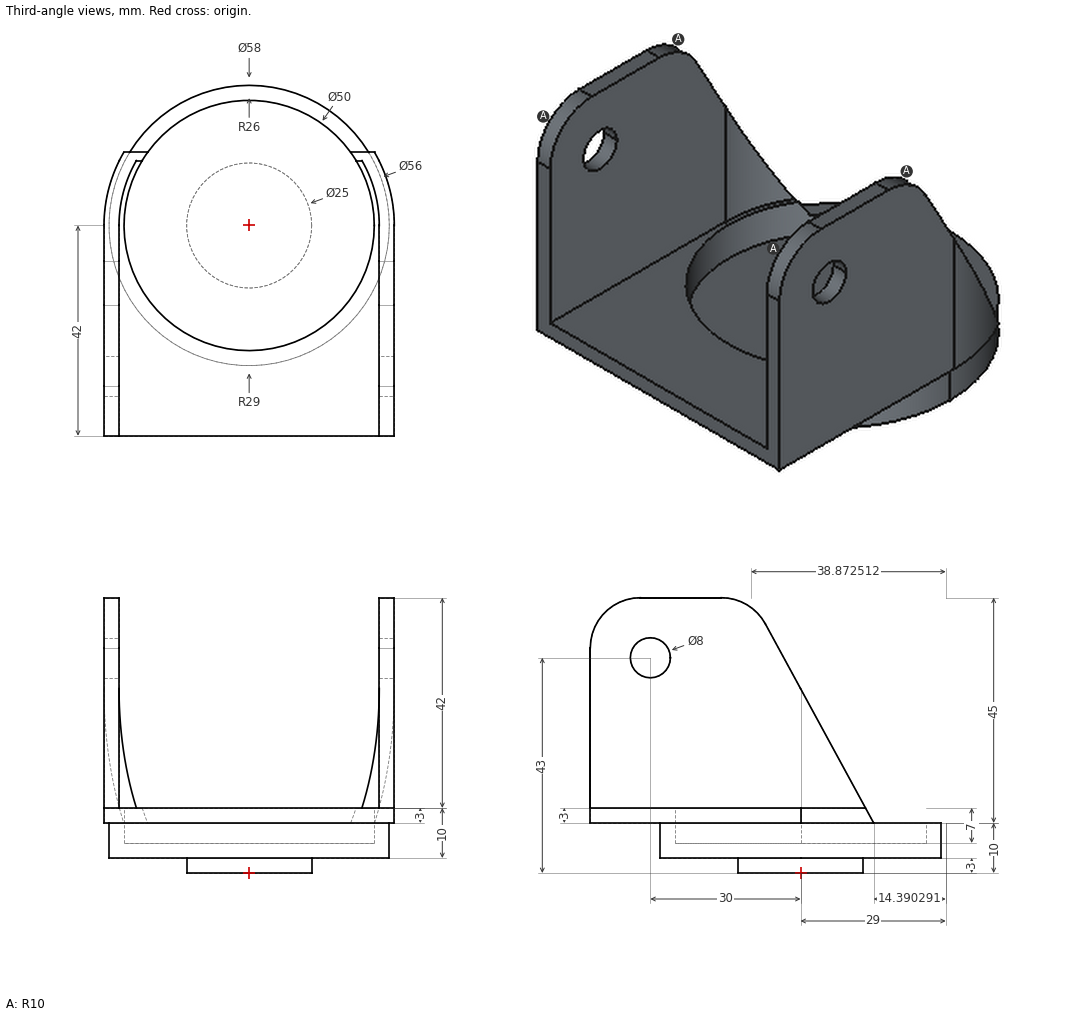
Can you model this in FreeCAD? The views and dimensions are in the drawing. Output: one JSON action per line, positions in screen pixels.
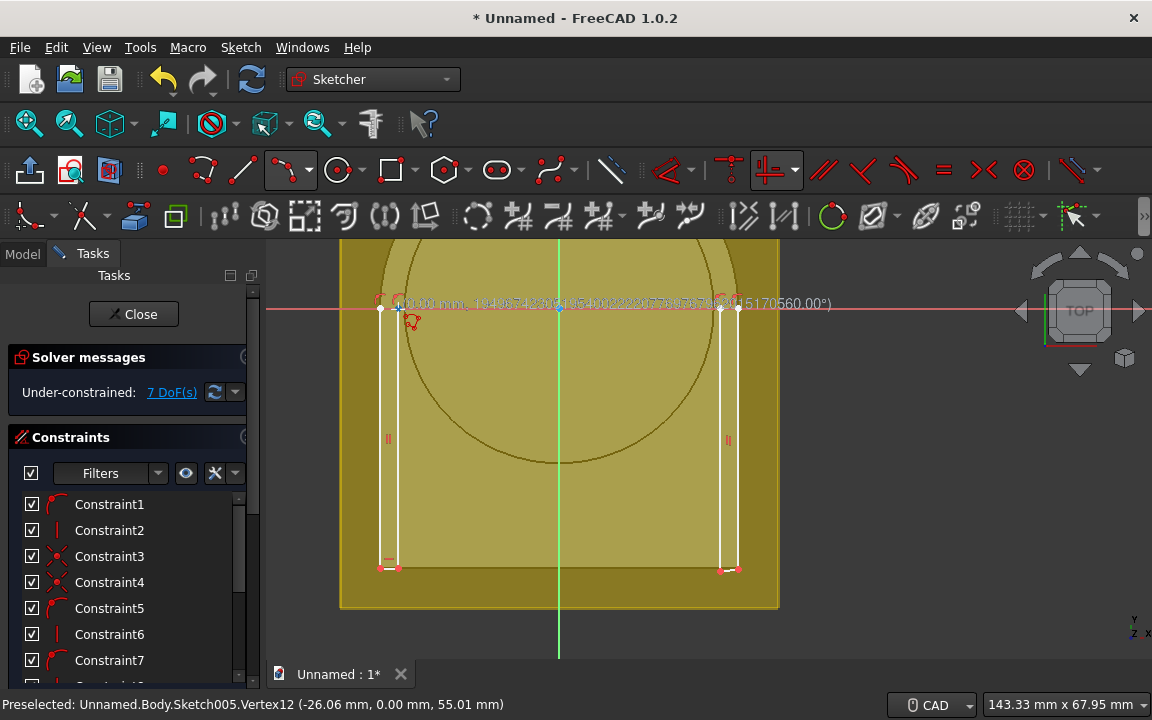
{"action": "left_click", "coordinate": [284, 170]}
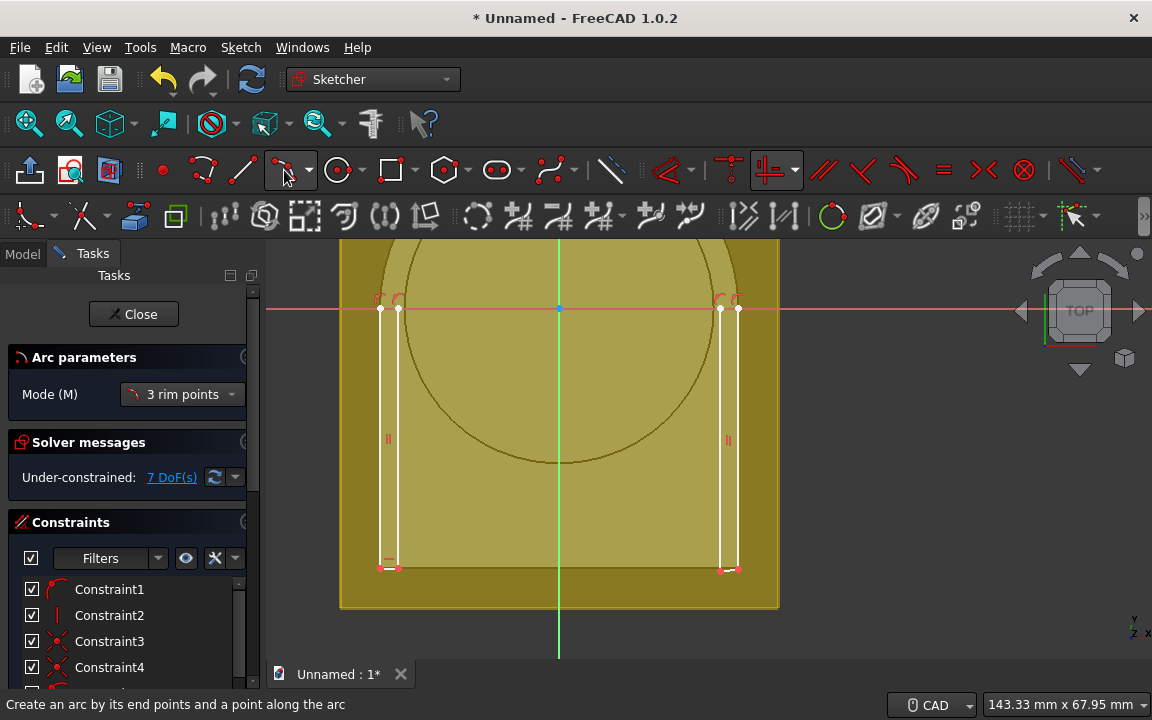
{"action": "left_click", "coordinate": [738, 309]}
{"action": "left_click", "coordinate": [380, 309]}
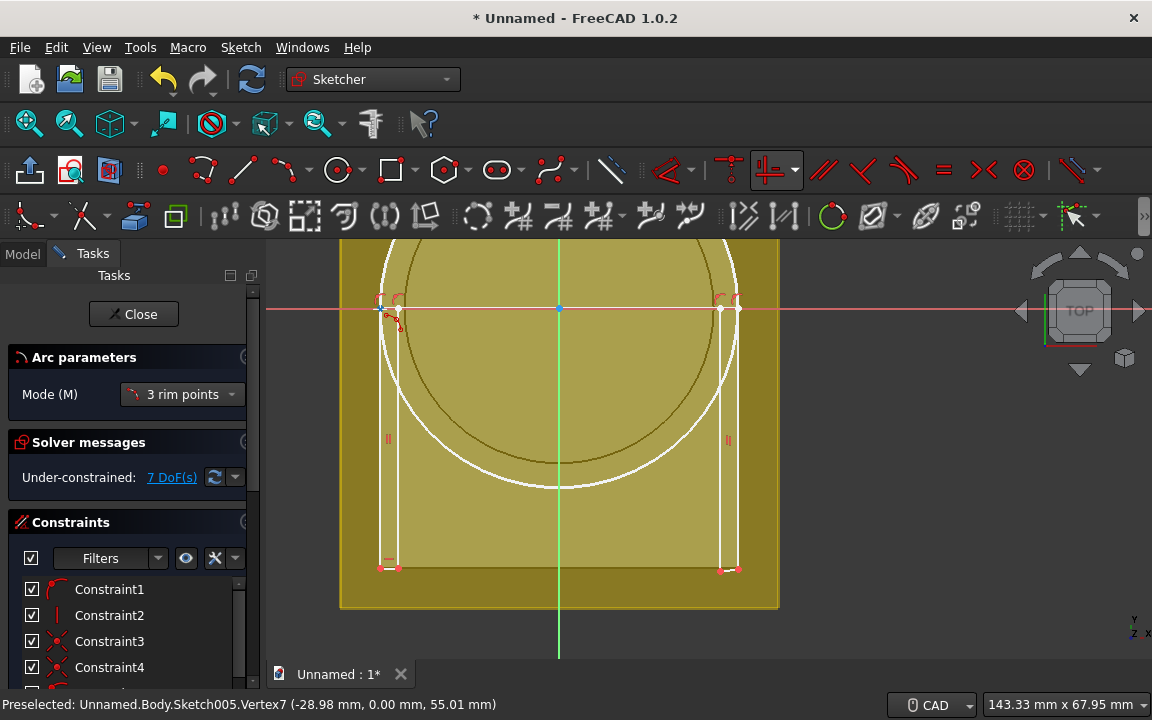
{"action": "scroll", "coordinate": [740, 571], "scroll_direction": "down", "scroll_amount": 3}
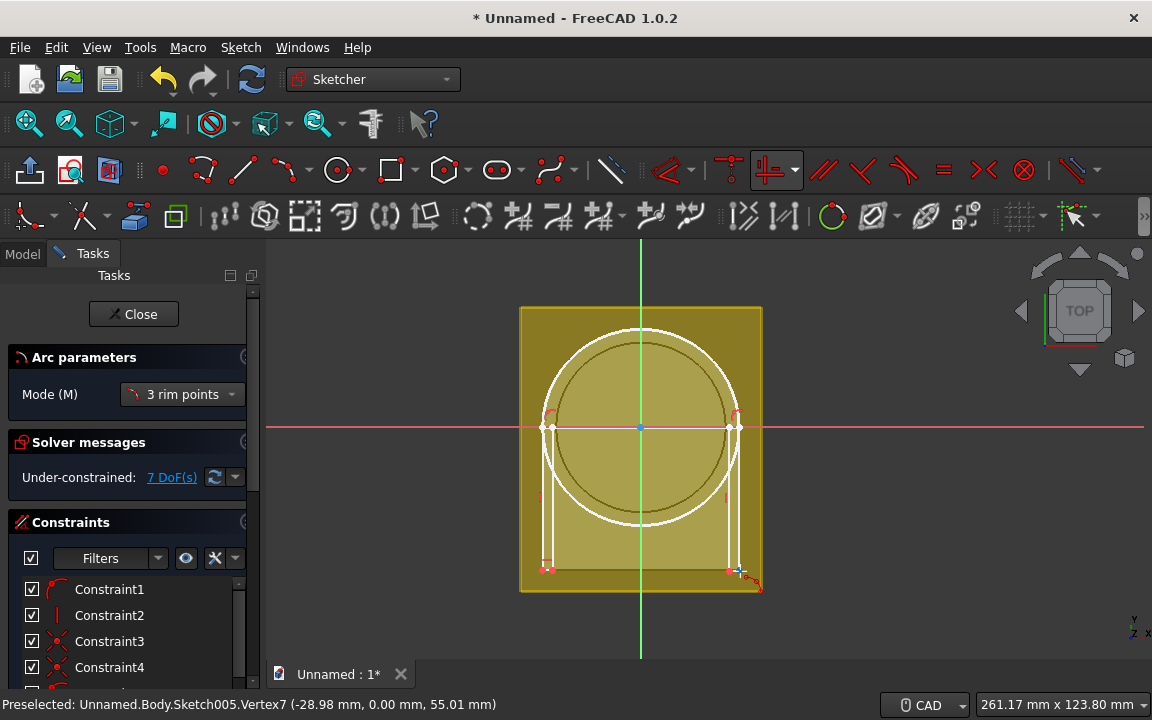
{"action": "left_click", "coordinate": [671, 334]}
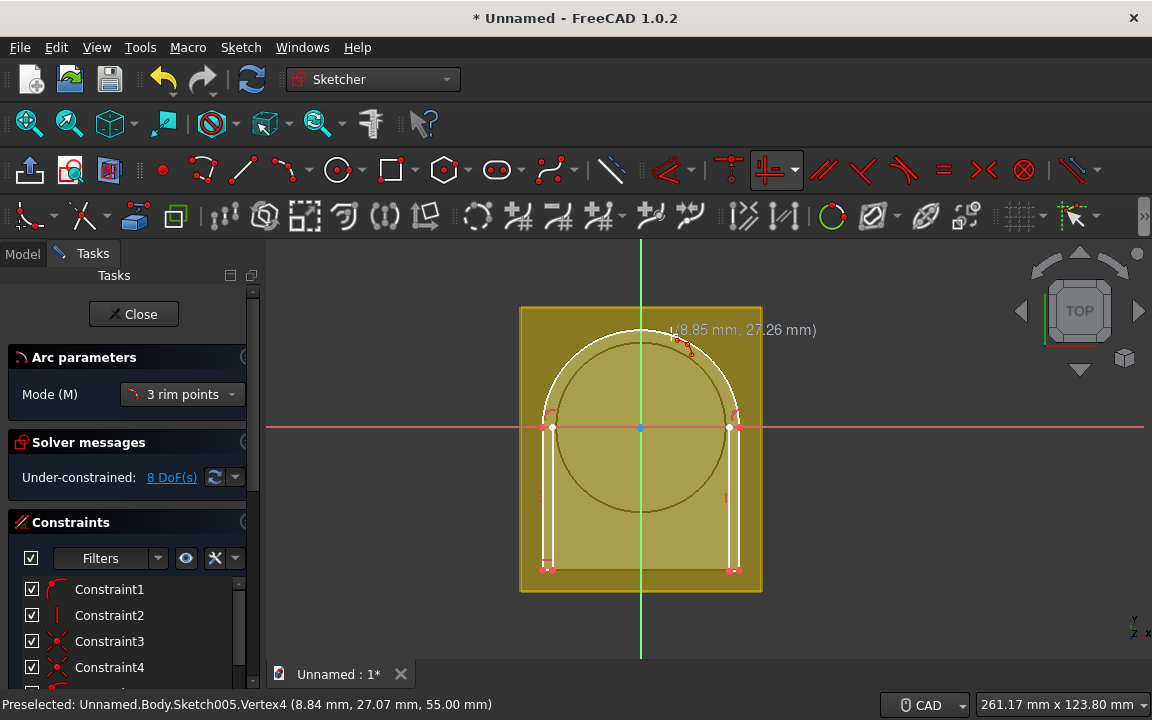
{"action": "scroll", "coordinate": [553, 427], "scroll_direction": "up", "scroll_amount": 3}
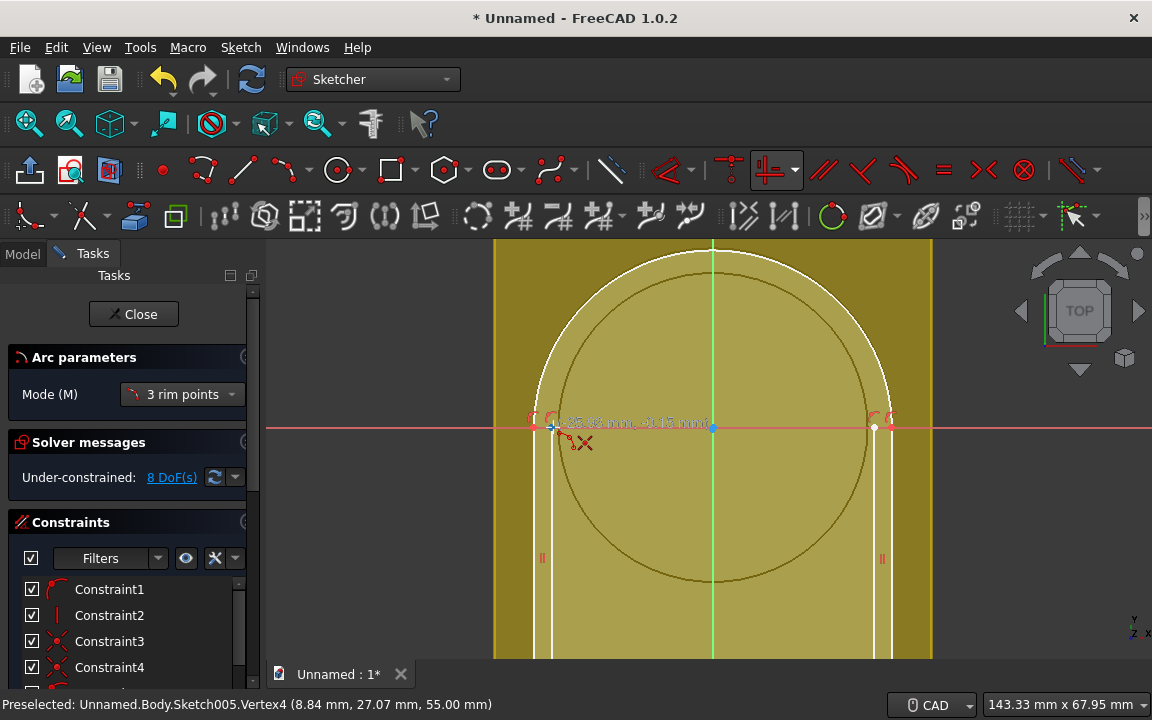
{"action": "left_click", "coordinate": [552, 427]}
{"action": "left_click", "coordinate": [874, 427]}
{"action": "left_click", "coordinate": [619, 297]}
{"action": "key", "text": "Escape"}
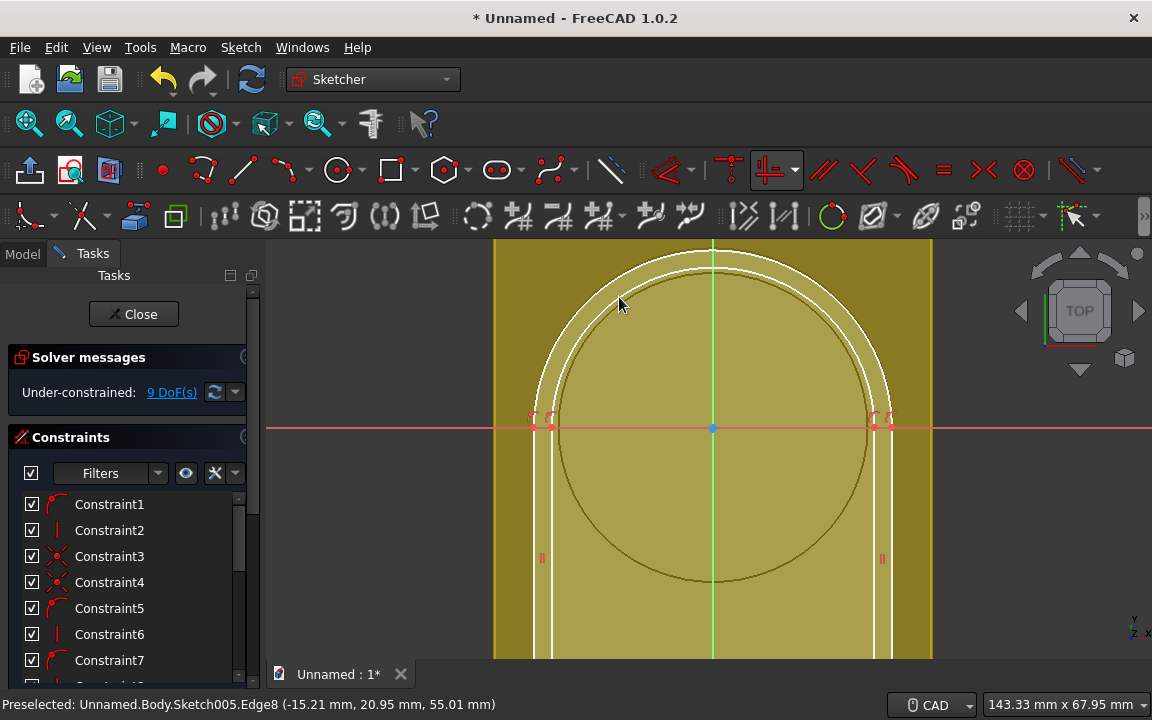
{"action": "left_click", "coordinate": [874, 506]}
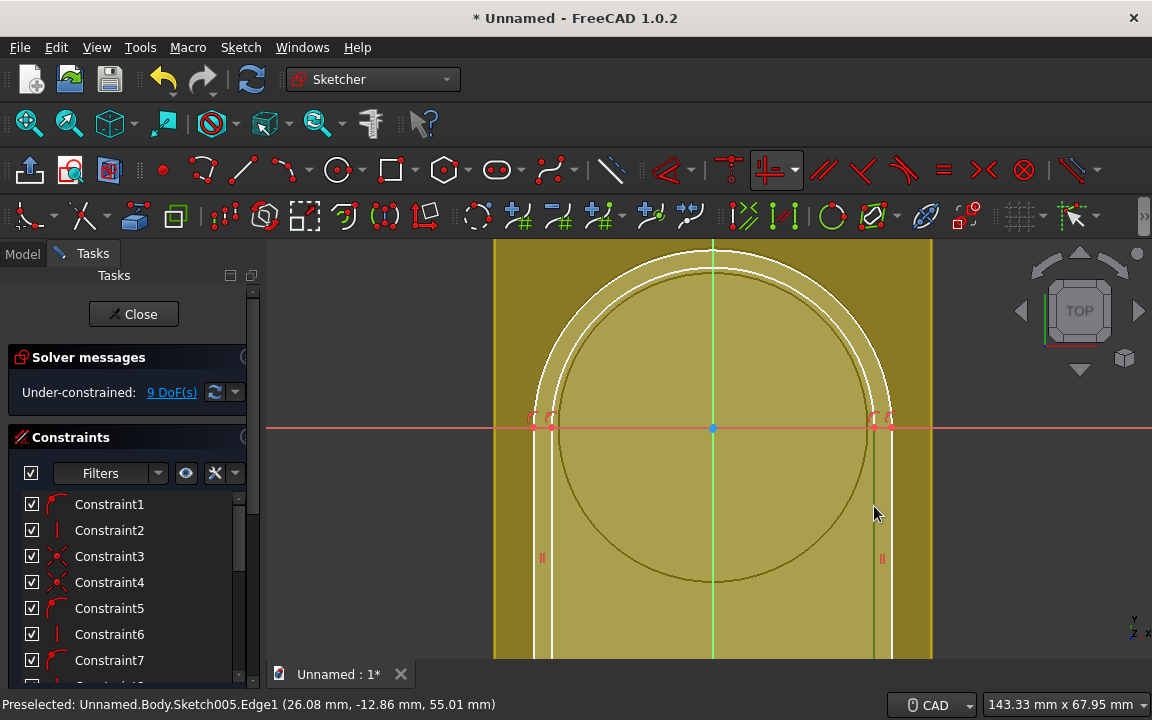
{"action": "left_click", "coordinate": [807, 298]}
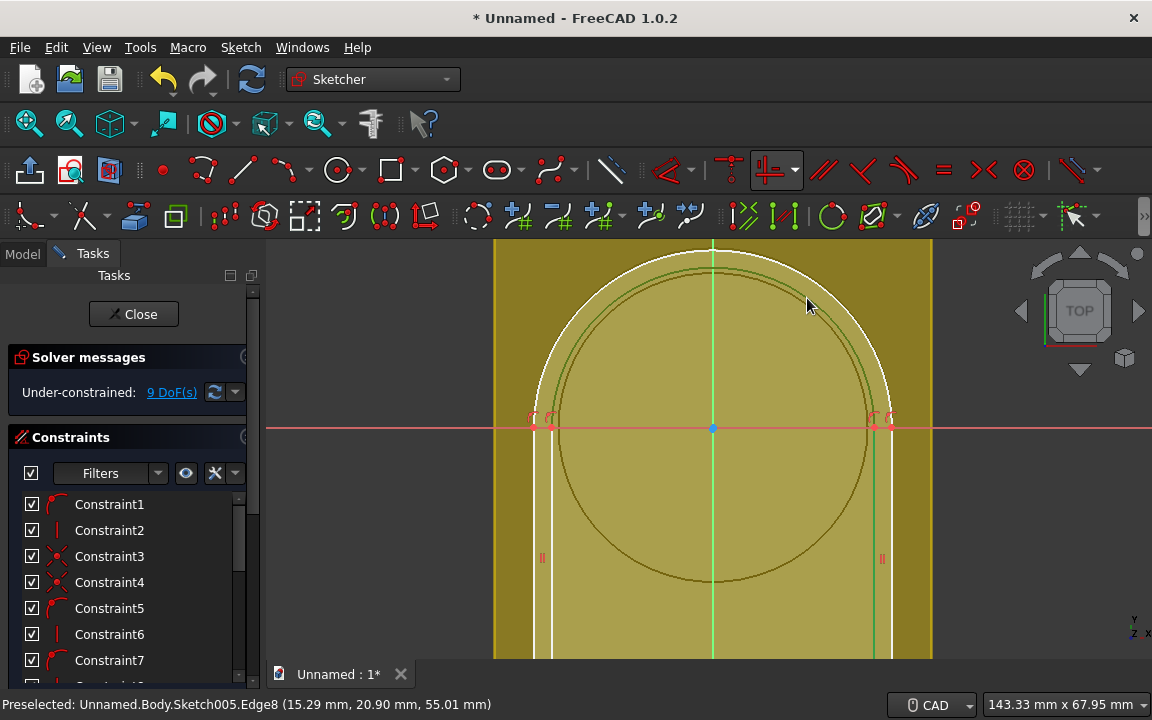
{"action": "left_click", "coordinate": [904, 170]}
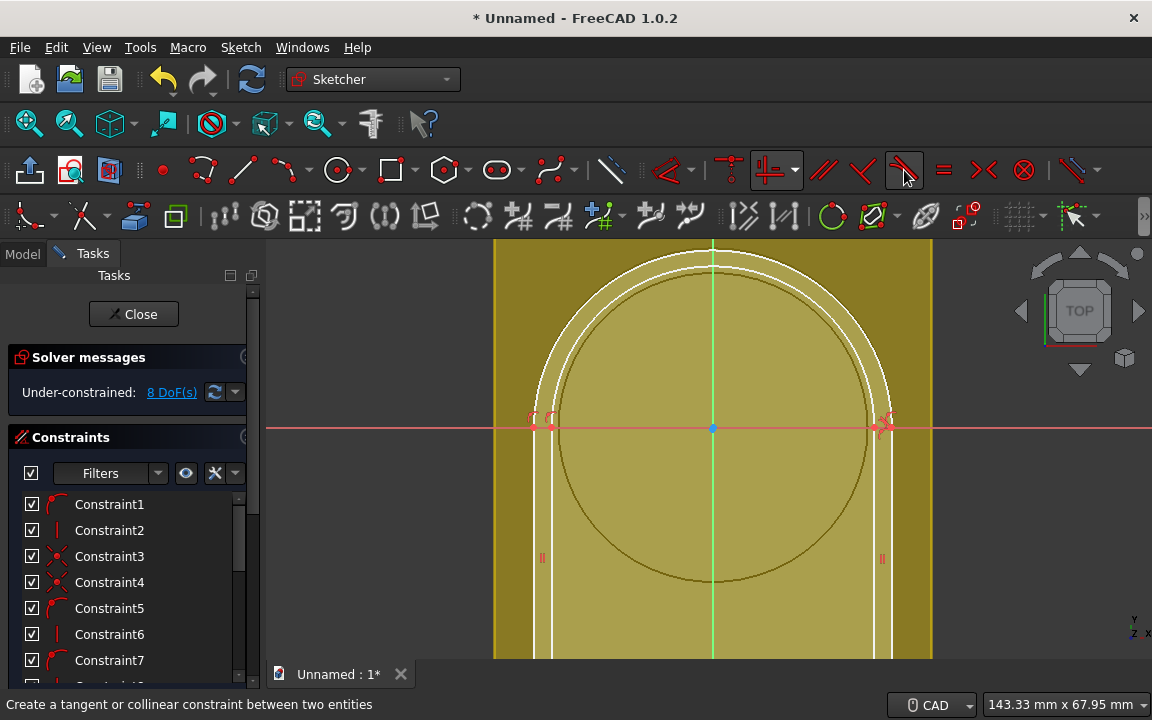
{"action": "scroll", "coordinate": [552, 426], "scroll_direction": "down", "scroll_amount": 3}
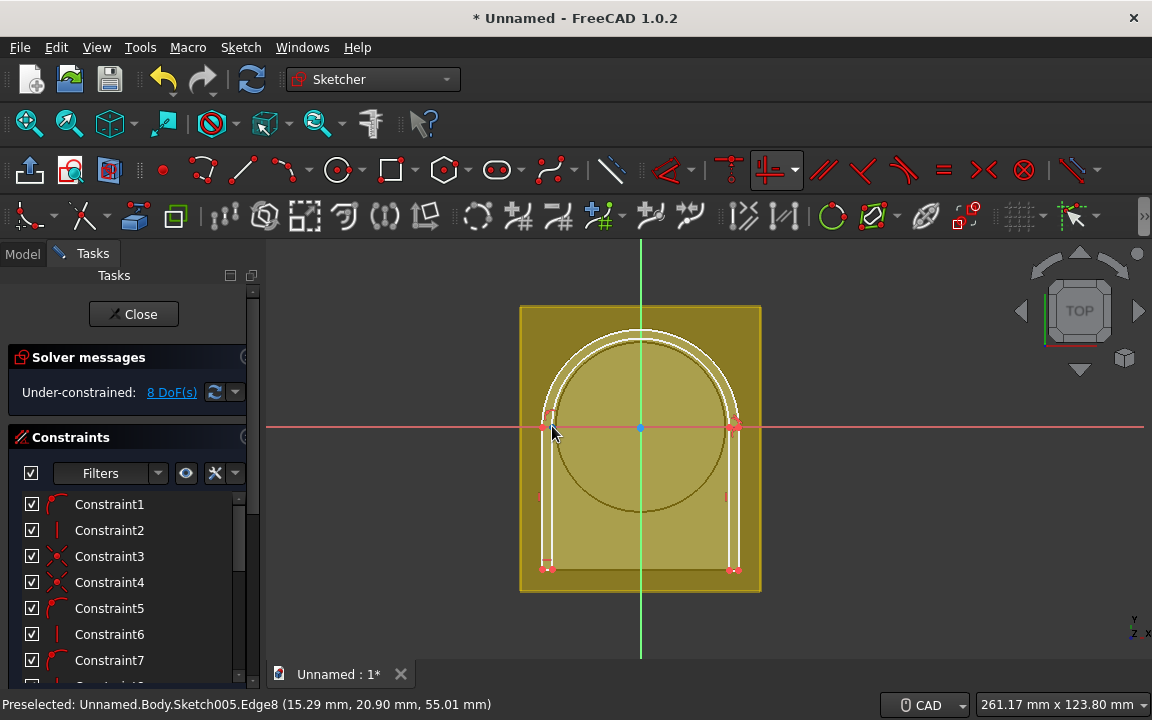
{"action": "scroll", "coordinate": [734, 571], "scroll_direction": "up", "scroll_amount": 6}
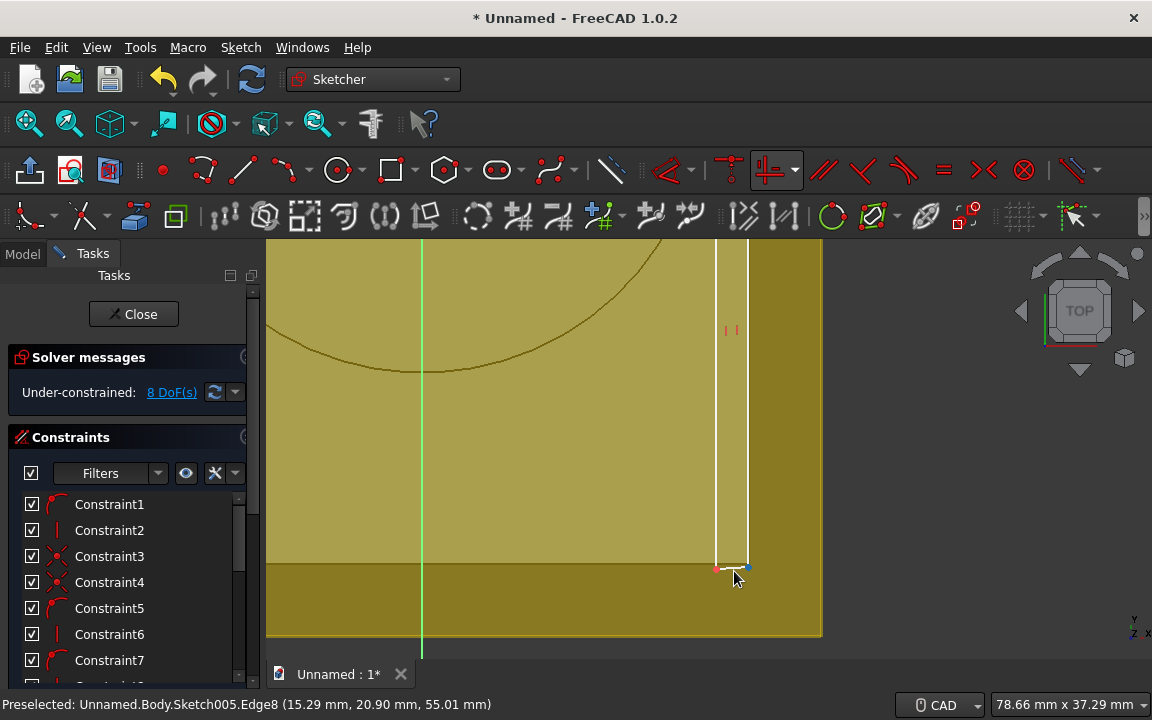
{"action": "left_click", "coordinate": [732, 568]}